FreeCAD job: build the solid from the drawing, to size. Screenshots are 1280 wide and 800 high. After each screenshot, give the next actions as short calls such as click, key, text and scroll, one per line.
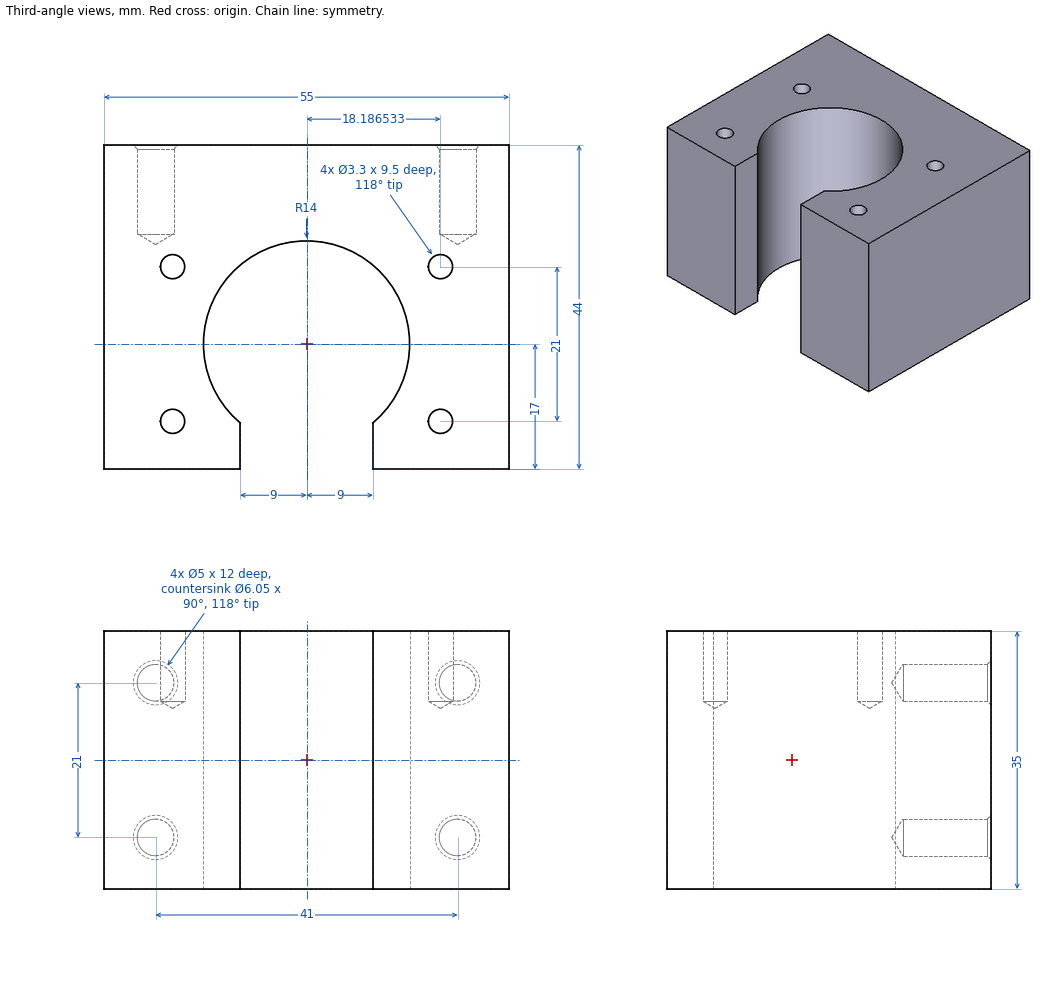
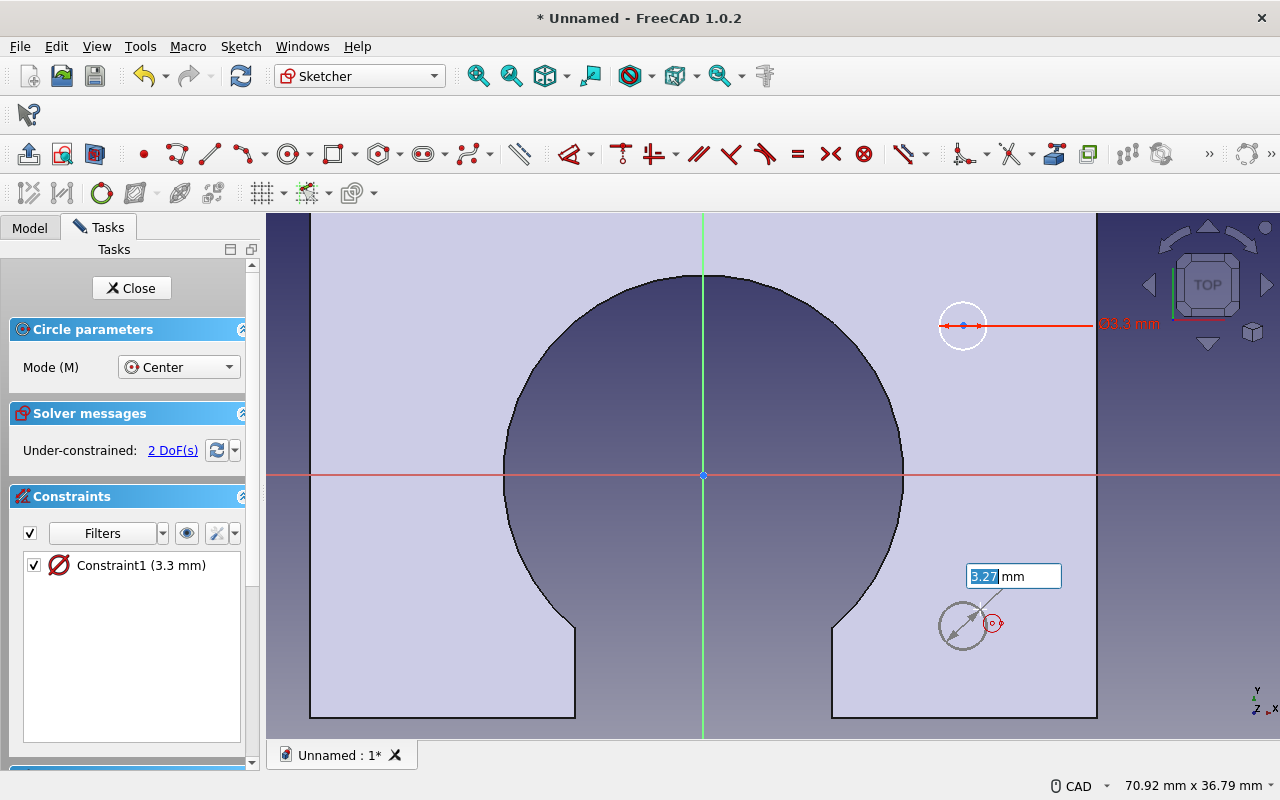
text(3.3)
key(Return)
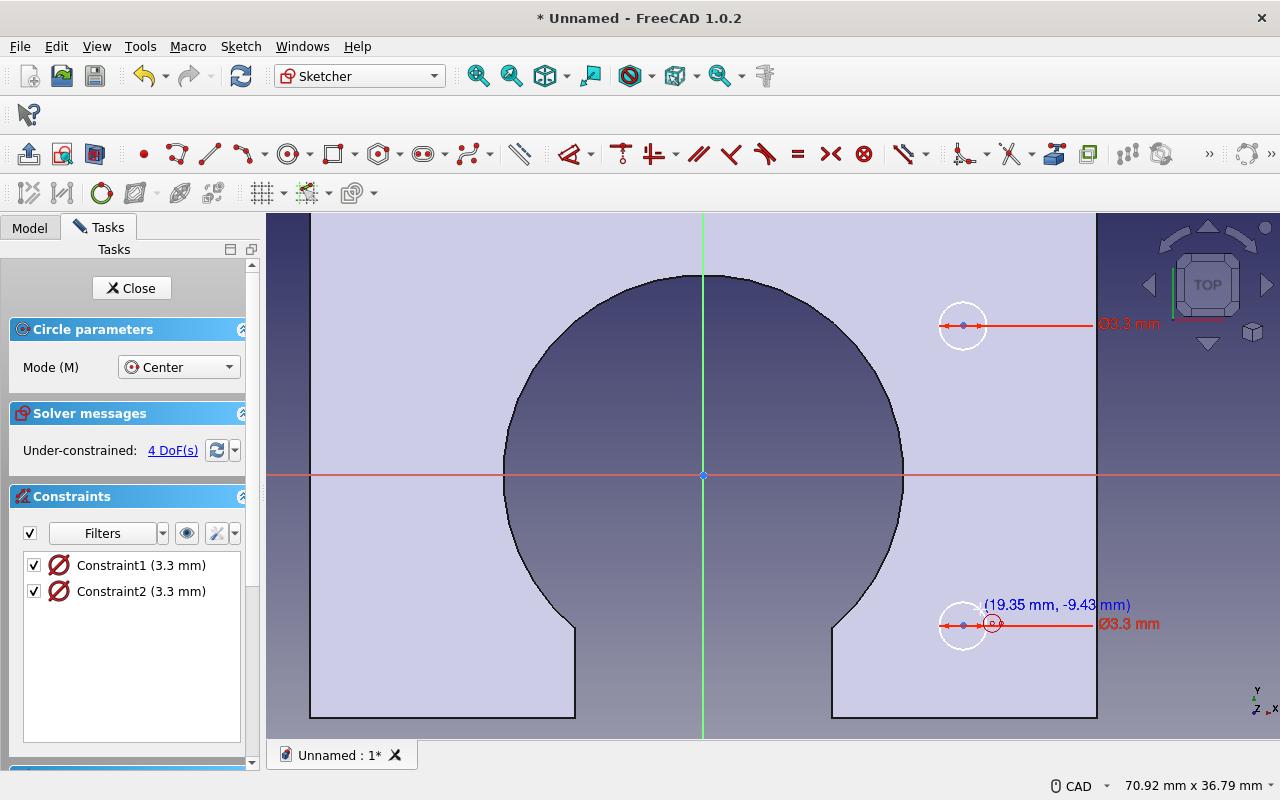
click(443, 625)
move(460, 609)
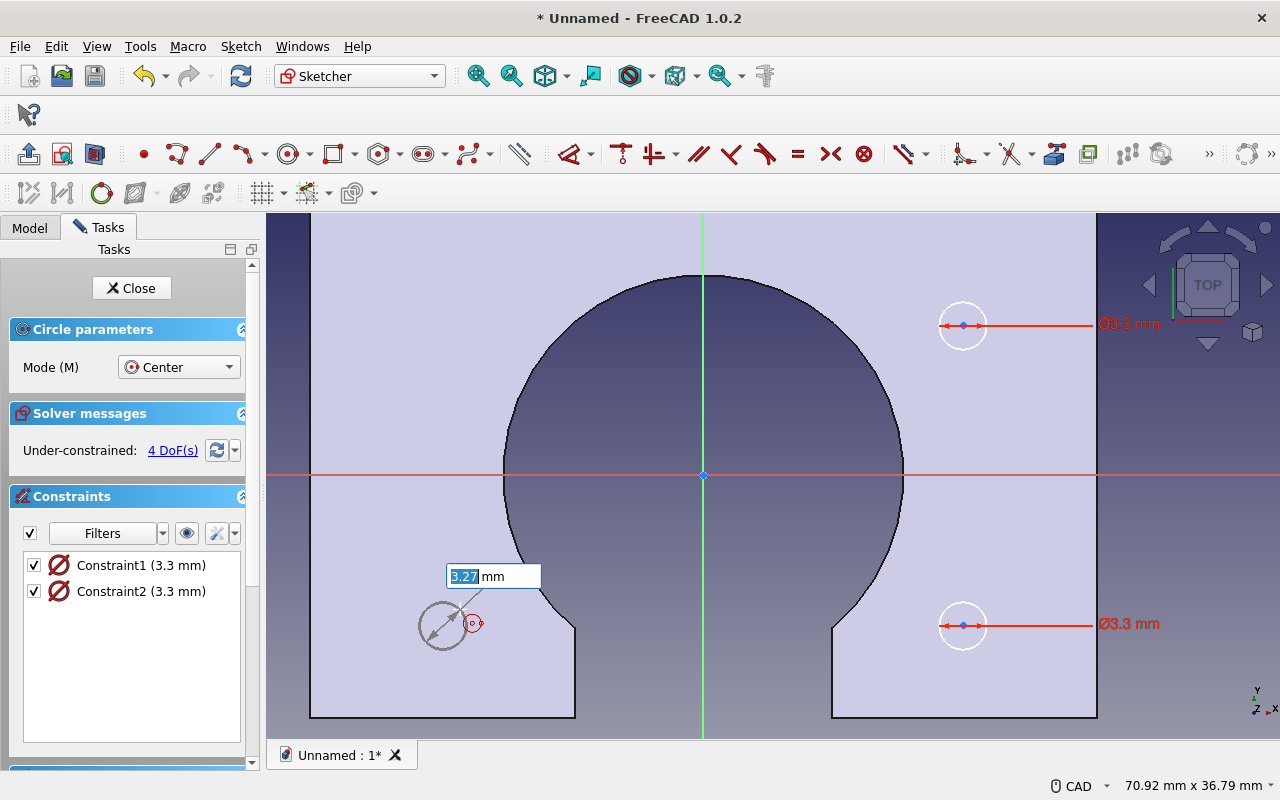
text(3.3)
key(Return)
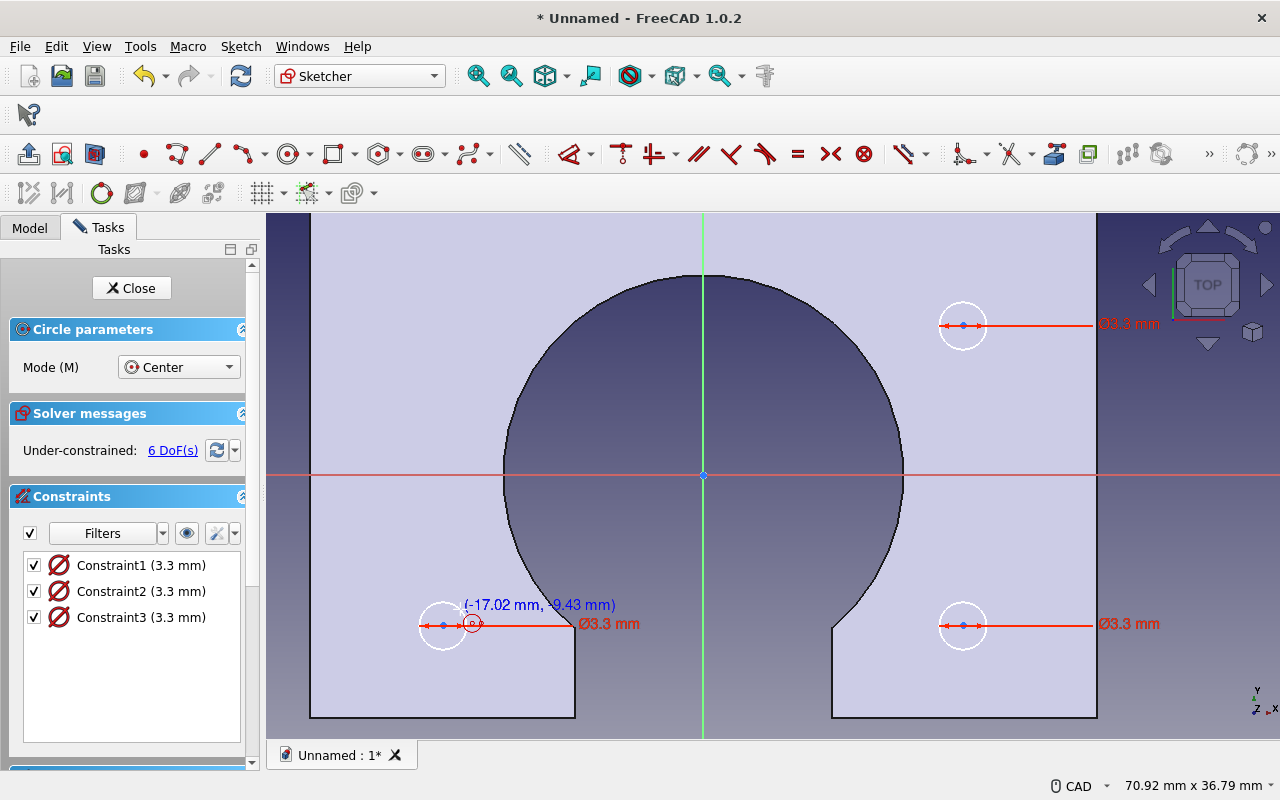
click(443, 325)
move(460, 308)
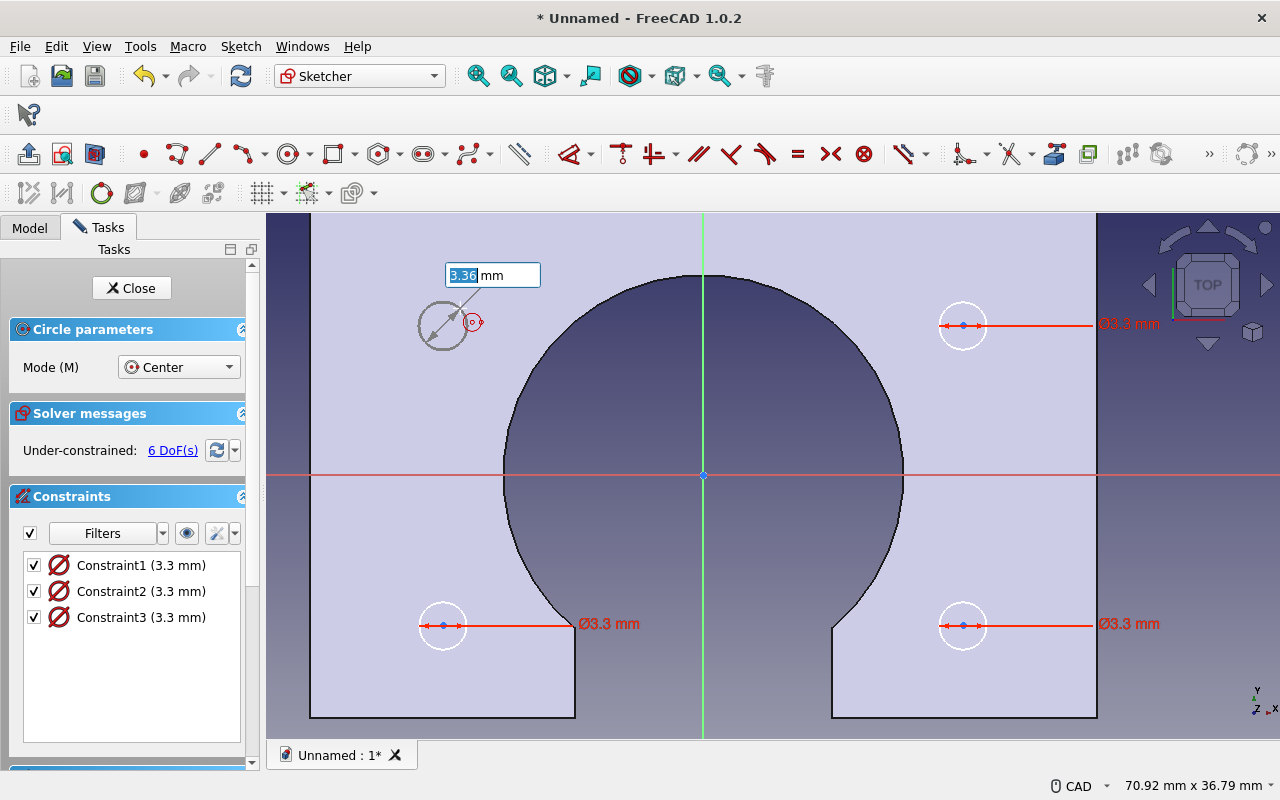
text(3.3)
key(Return)
key(Escape)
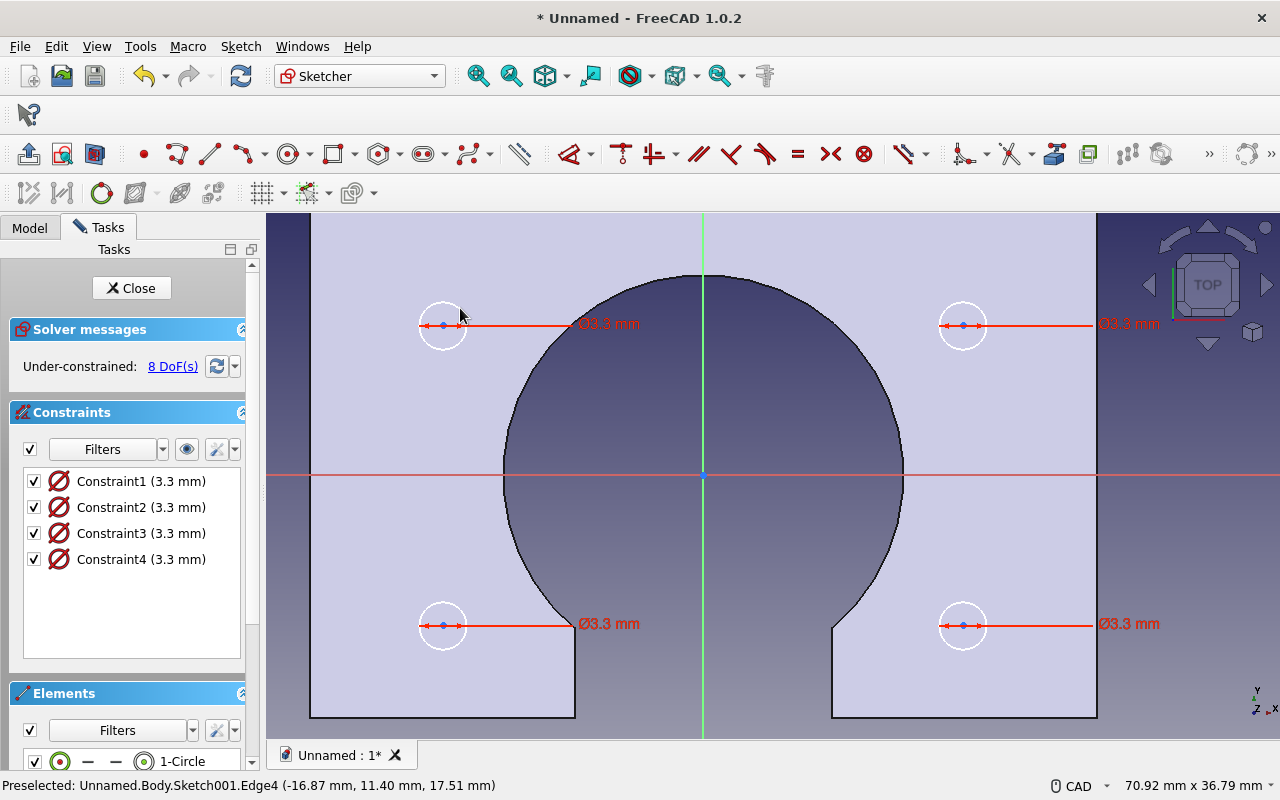
click(963, 326)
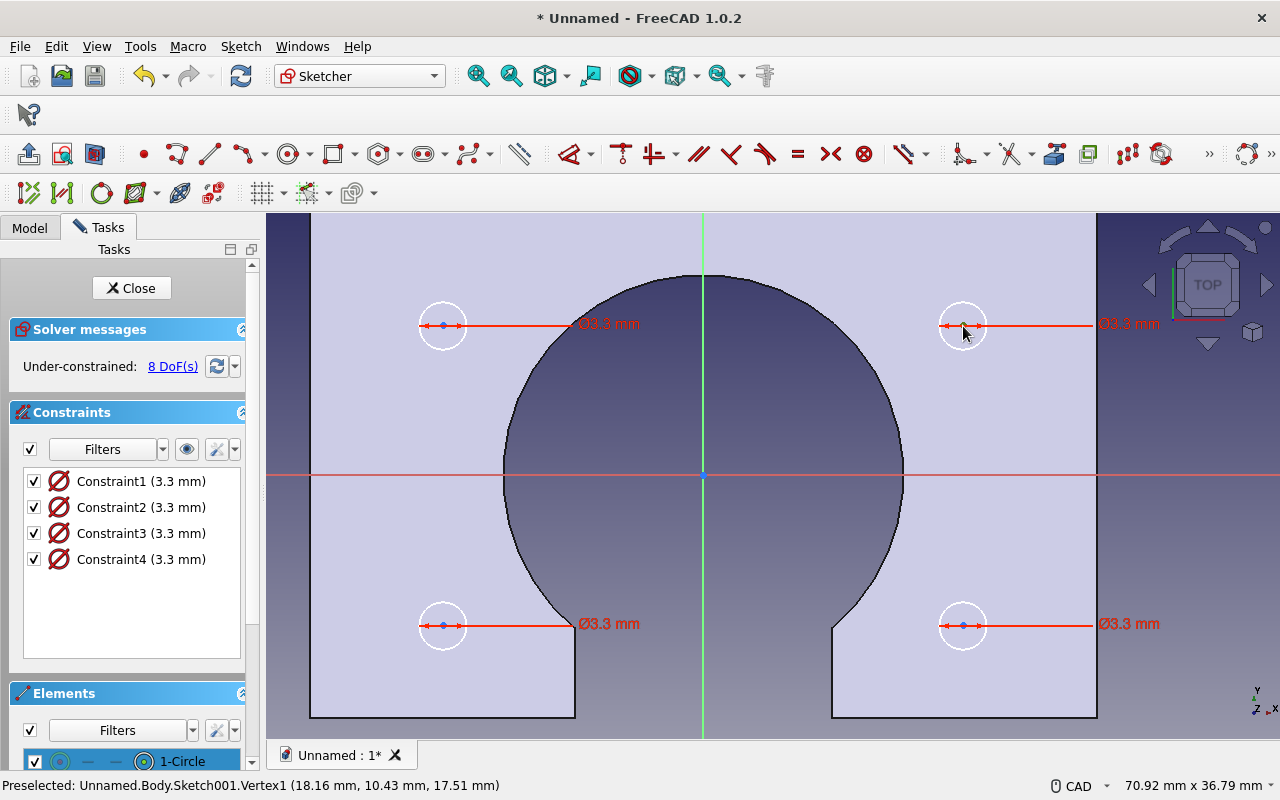
click(963, 626)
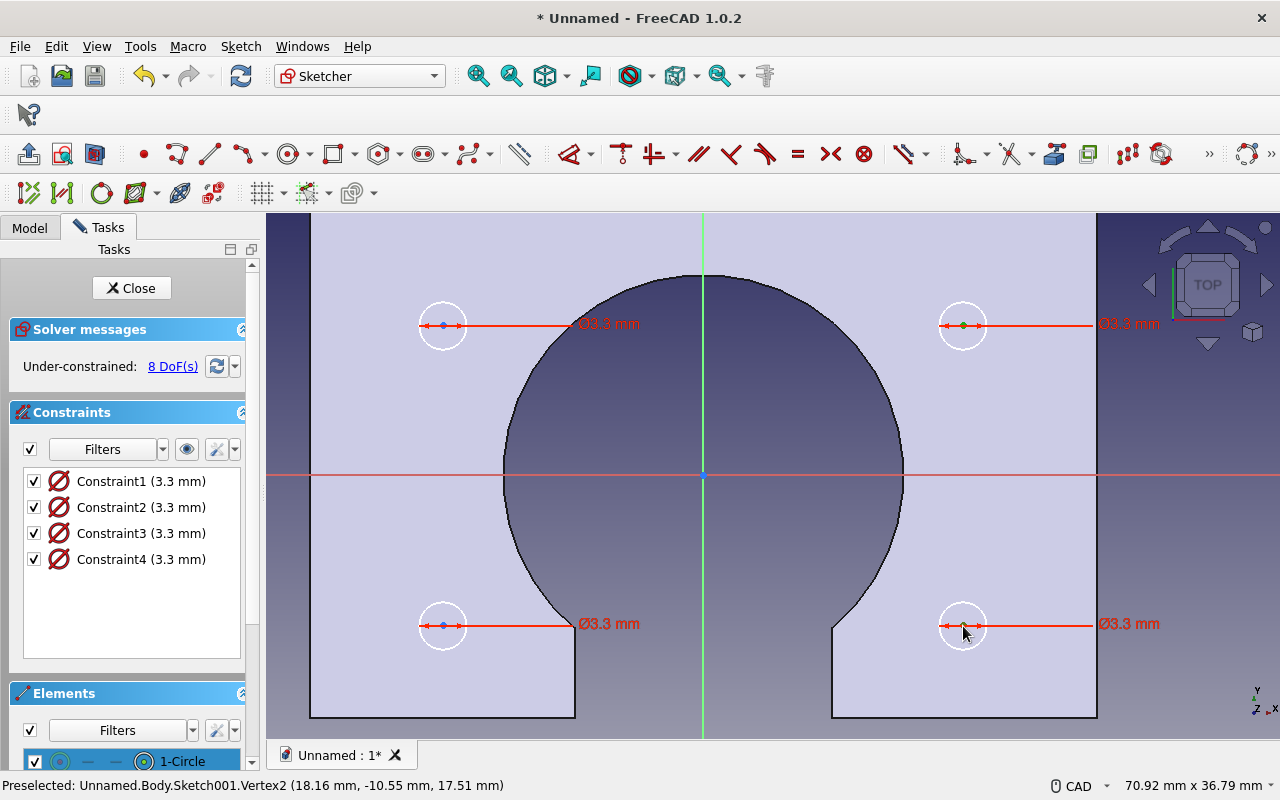
click(353, 475)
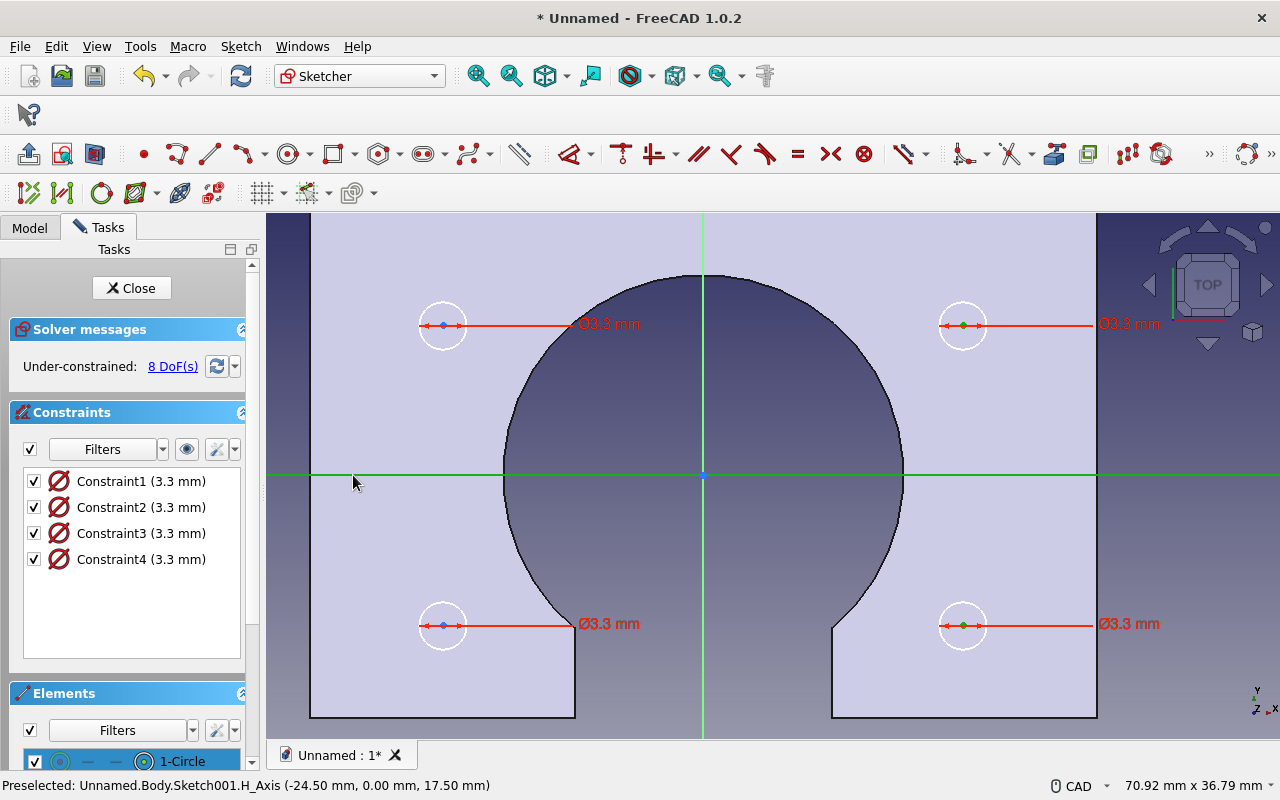
click(831, 154)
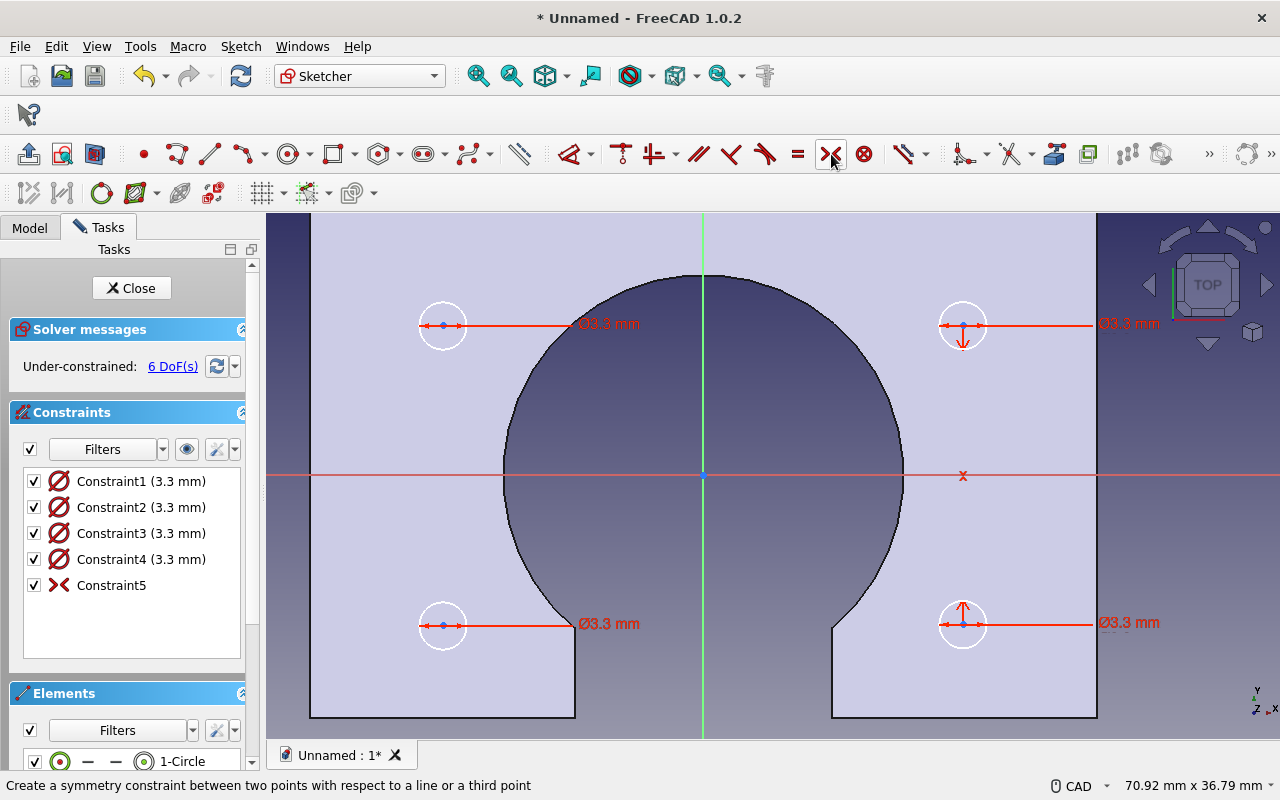
click(963, 625)